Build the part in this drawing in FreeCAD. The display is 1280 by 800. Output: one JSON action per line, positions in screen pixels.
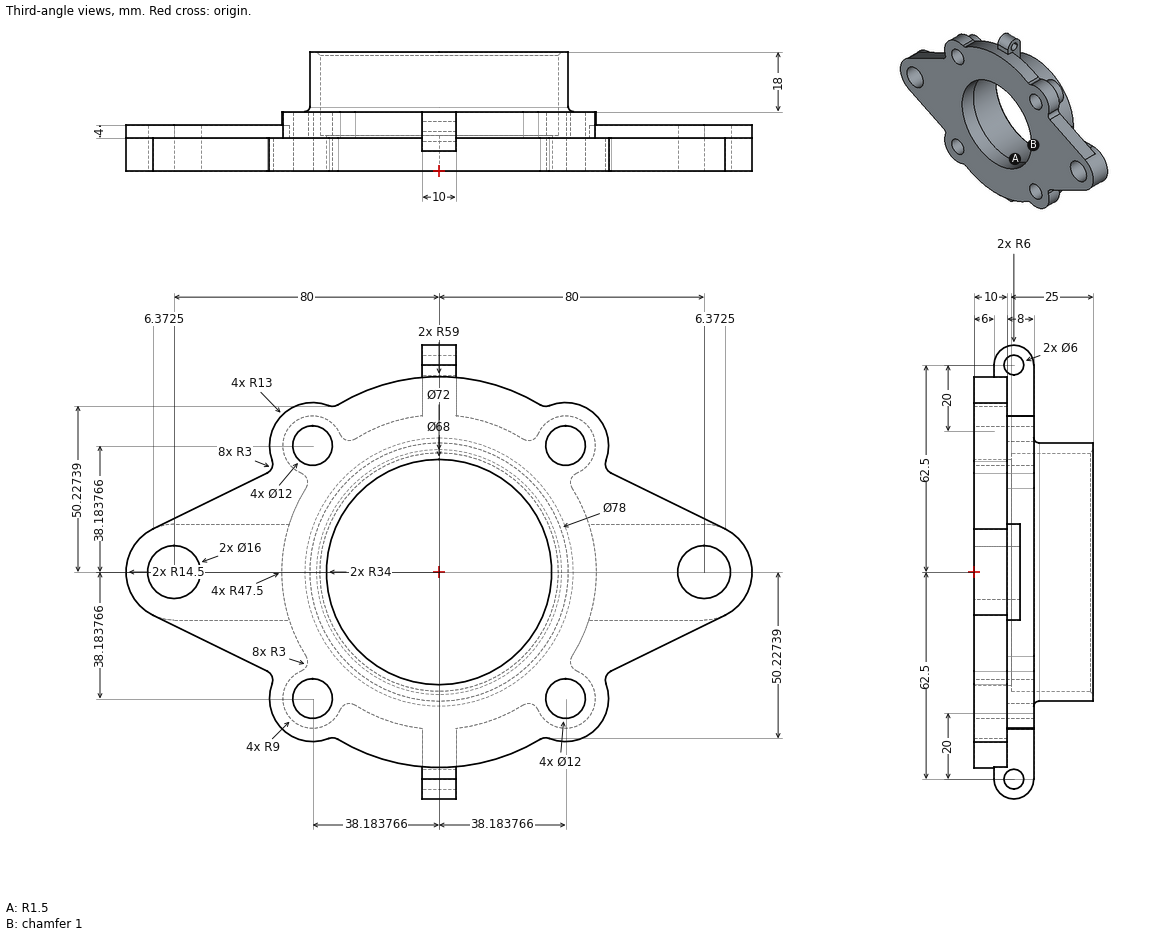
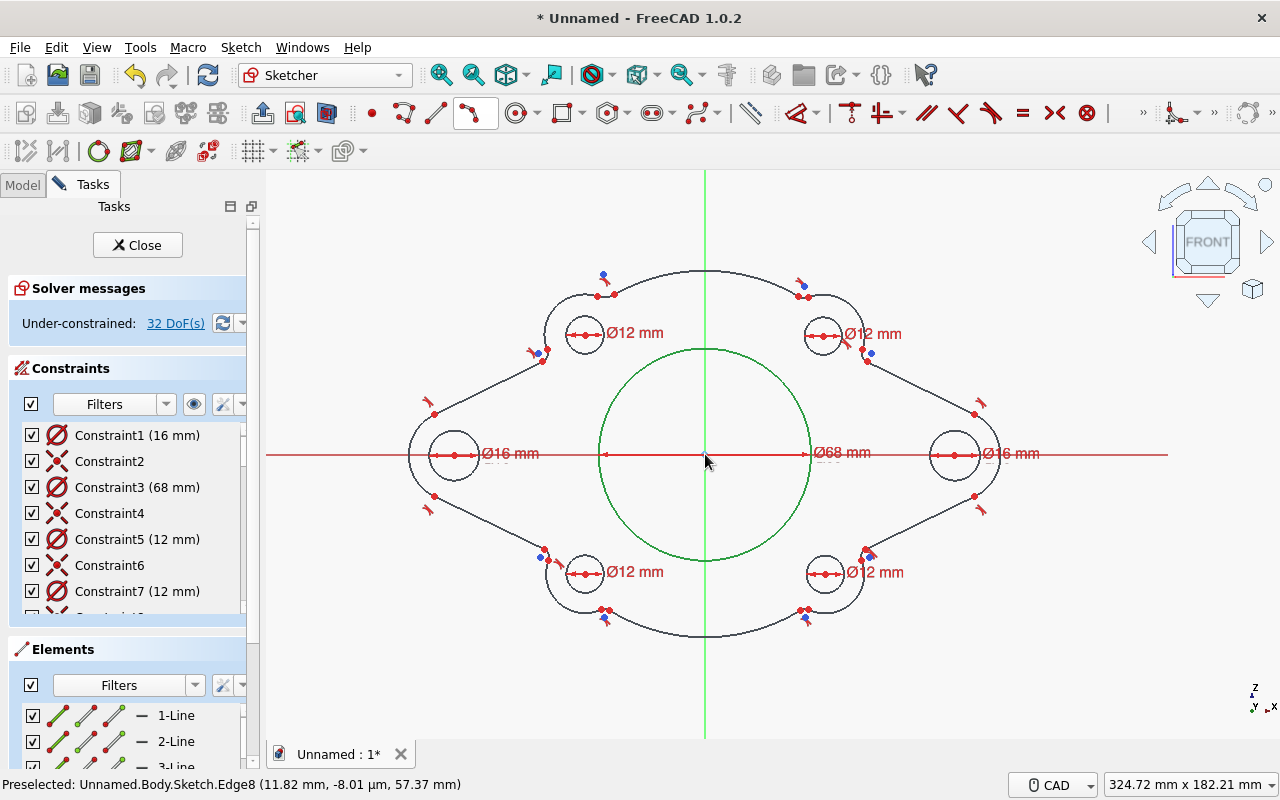
{"action": "scroll", "coordinate": [546, 359], "scroll_direction": "up", "scroll_amount": 6}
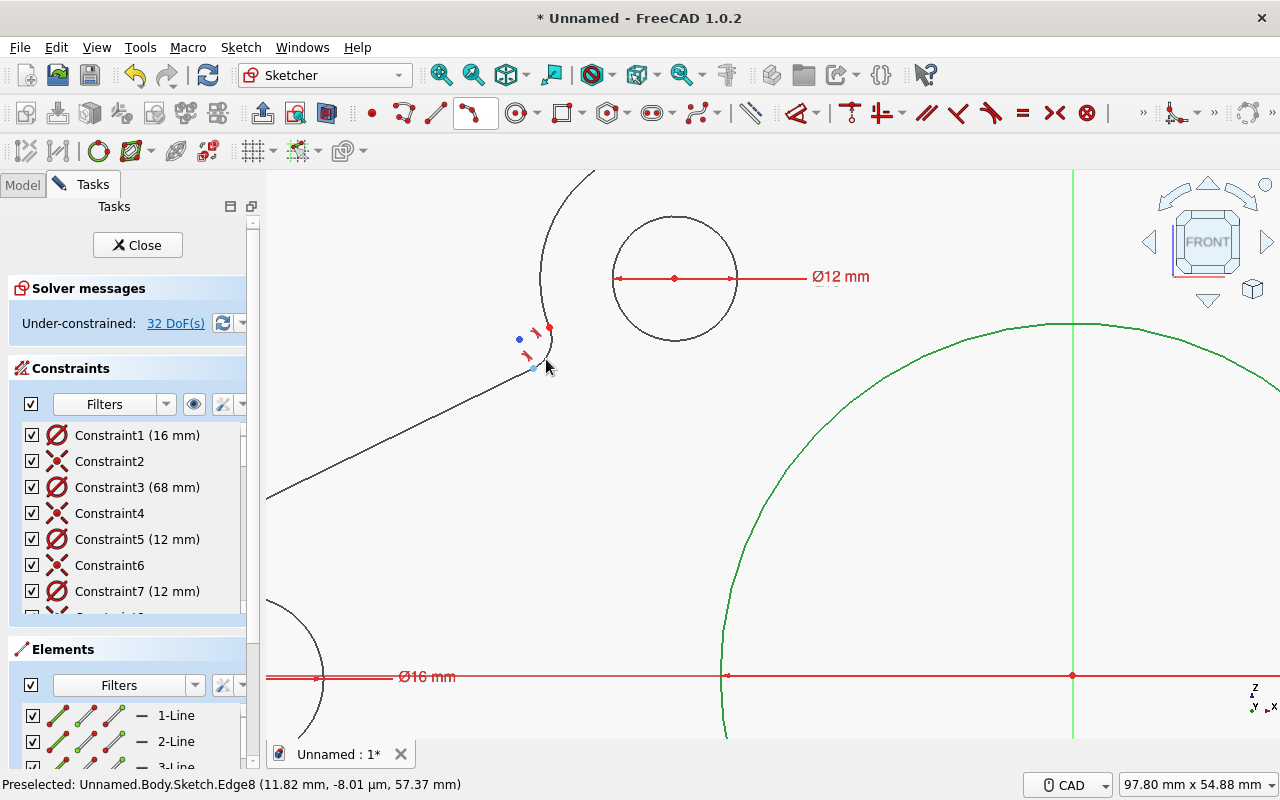
{"action": "left_click", "coordinate": [545, 359]}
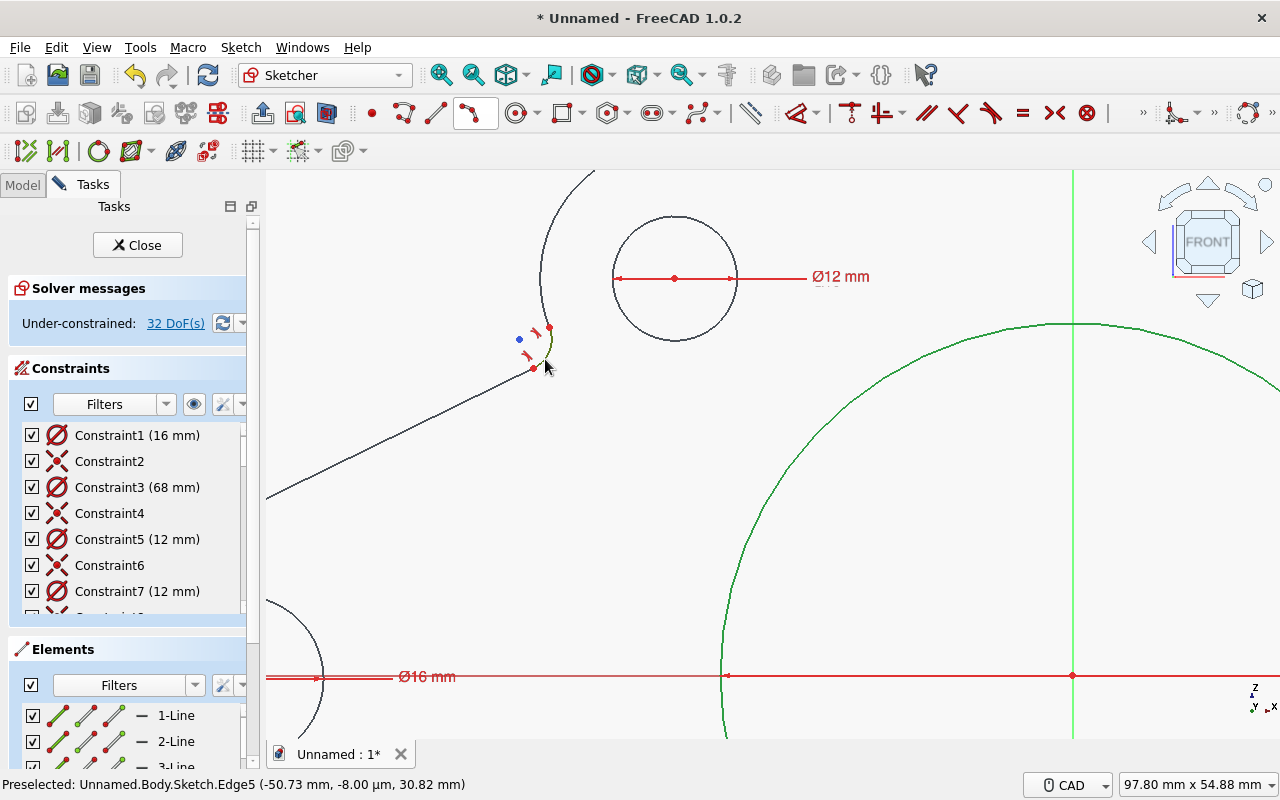
{"action": "scroll", "coordinate": [546, 359], "scroll_direction": "down", "scroll_amount": 6}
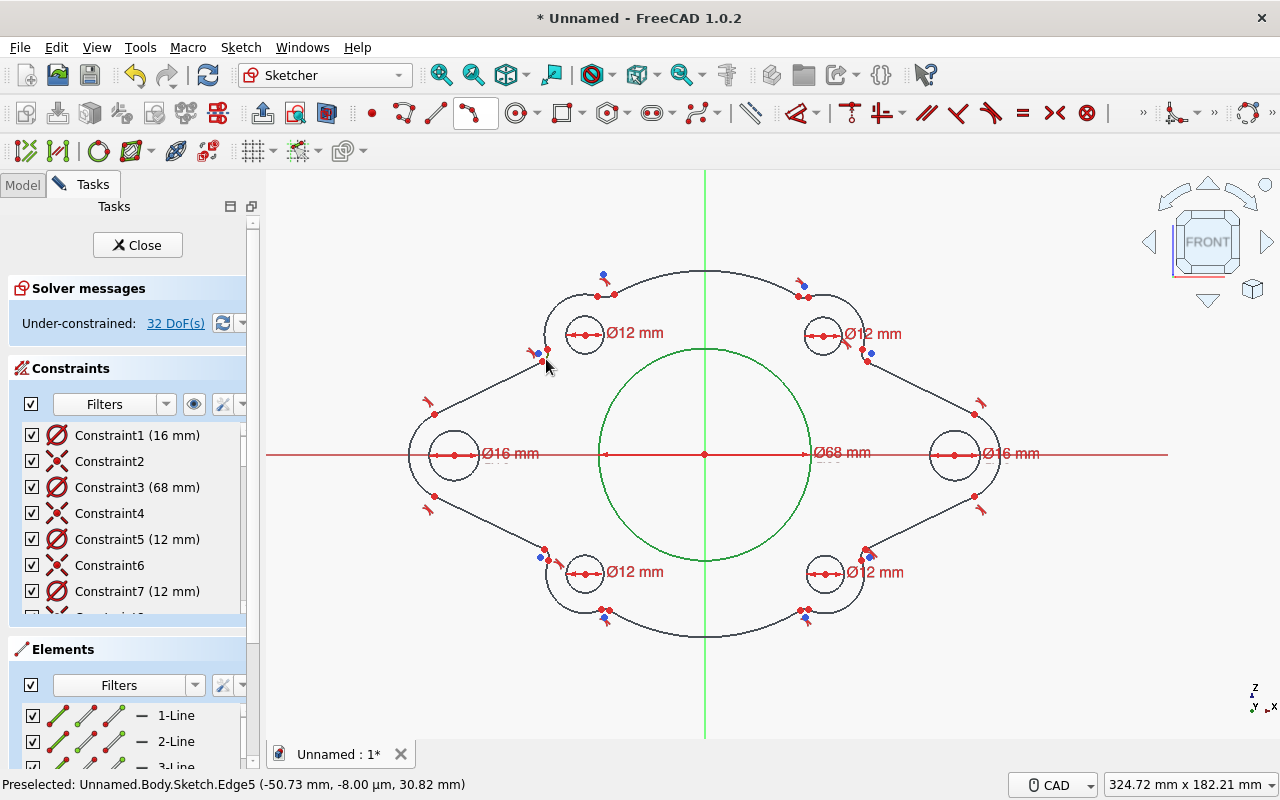
{"action": "scroll", "coordinate": [602, 297], "scroll_direction": "up", "scroll_amount": 5}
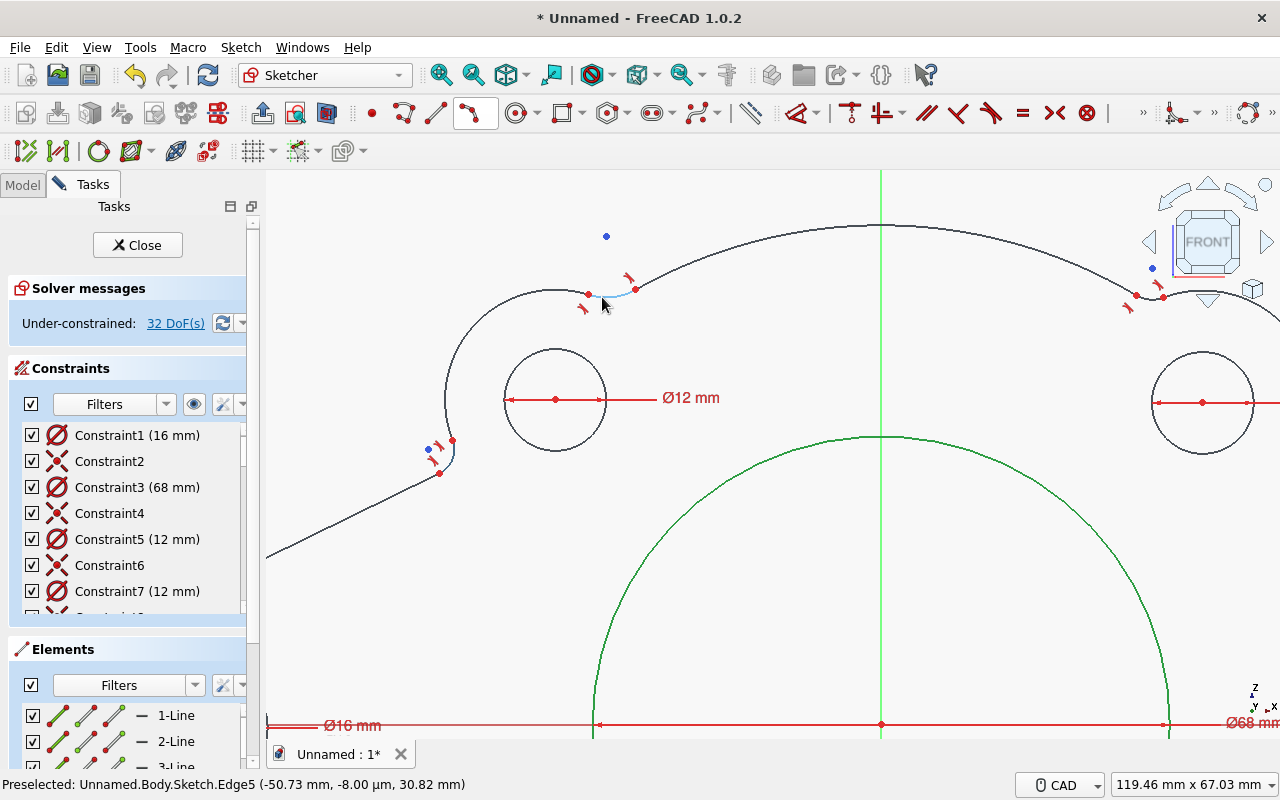
{"action": "left_click", "coordinate": [603, 297]}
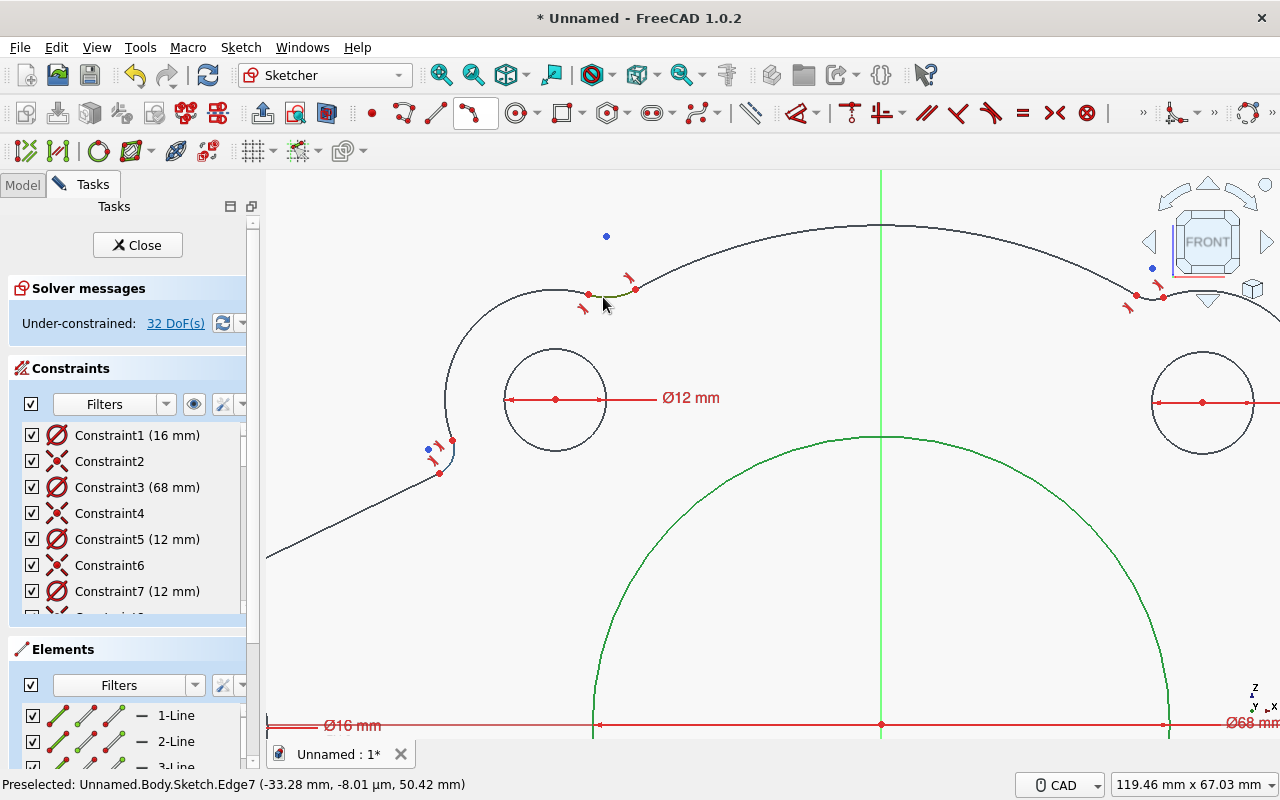
{"action": "scroll", "coordinate": [602, 297], "scroll_direction": "down", "scroll_amount": 5}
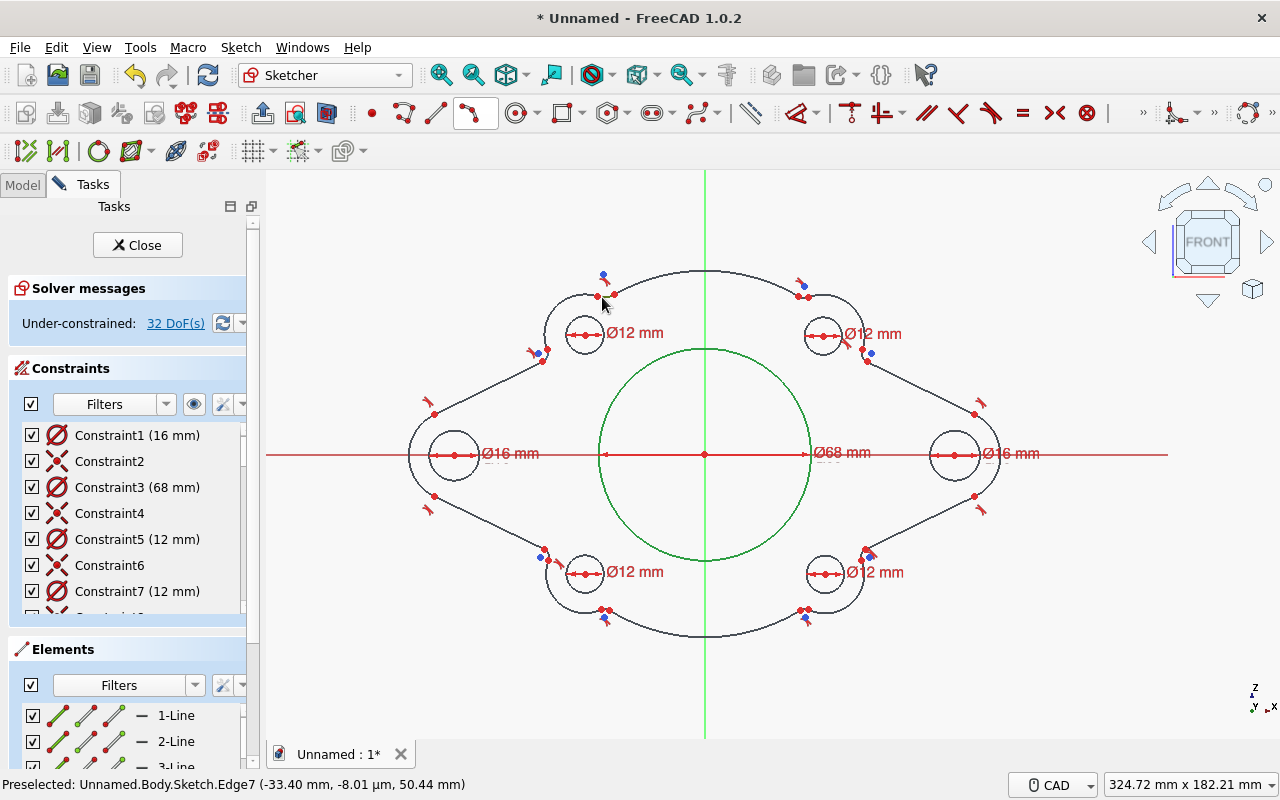
{"action": "scroll", "coordinate": [804, 298], "scroll_direction": "up", "scroll_amount": 5}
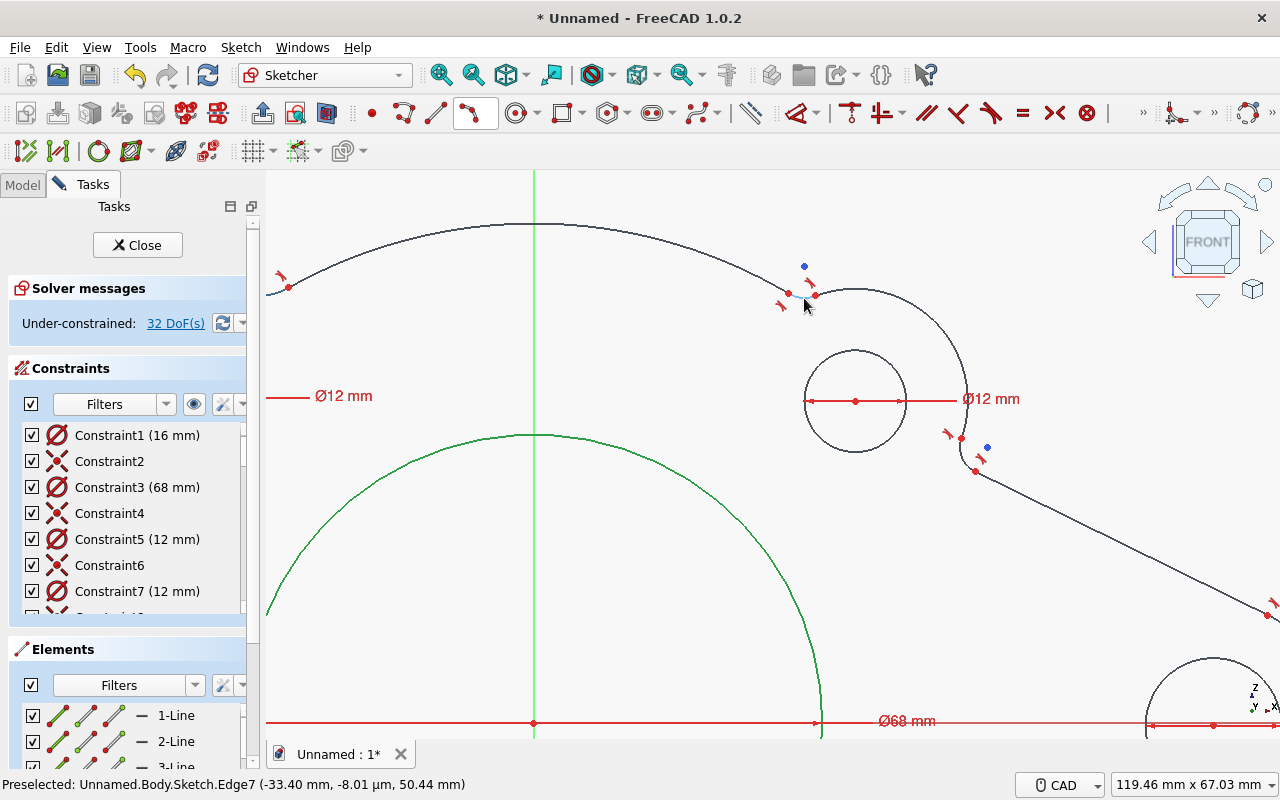
{"action": "left_click", "coordinate": [802, 298]}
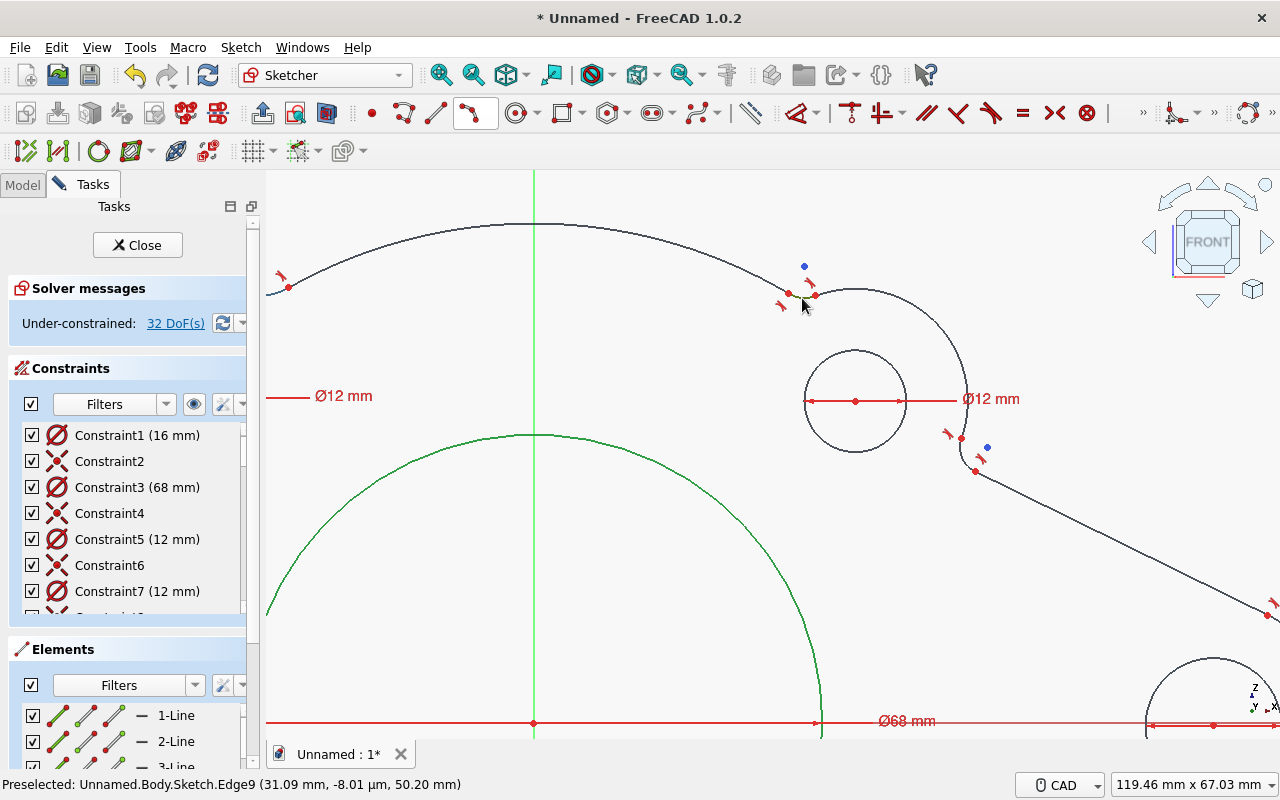
{"action": "left_click", "coordinate": [960, 450]}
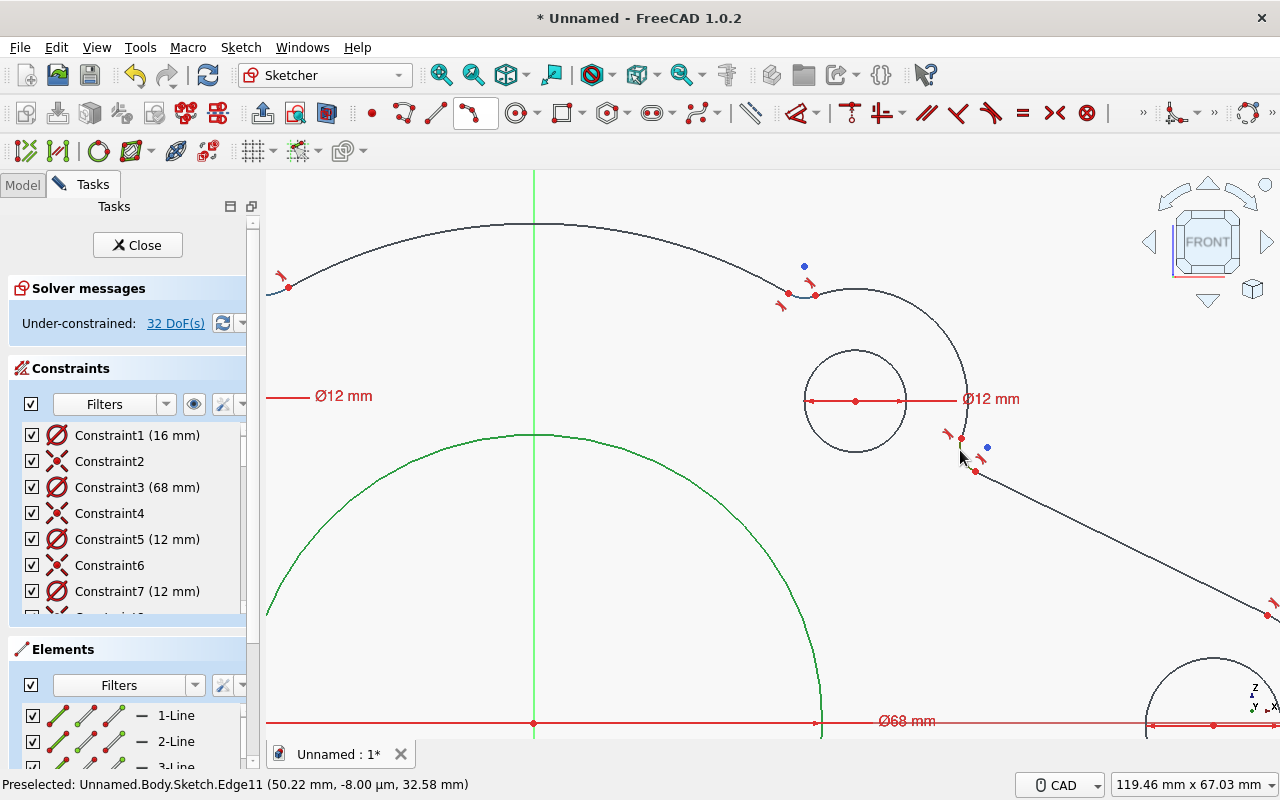
{"action": "scroll", "coordinate": [804, 298], "scroll_direction": "down", "scroll_amount": 5}